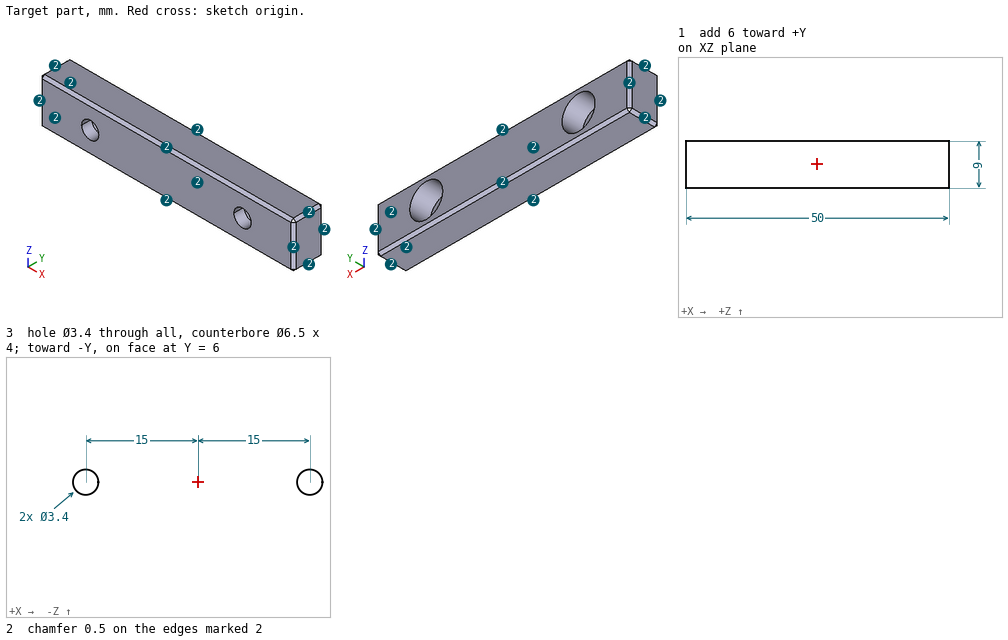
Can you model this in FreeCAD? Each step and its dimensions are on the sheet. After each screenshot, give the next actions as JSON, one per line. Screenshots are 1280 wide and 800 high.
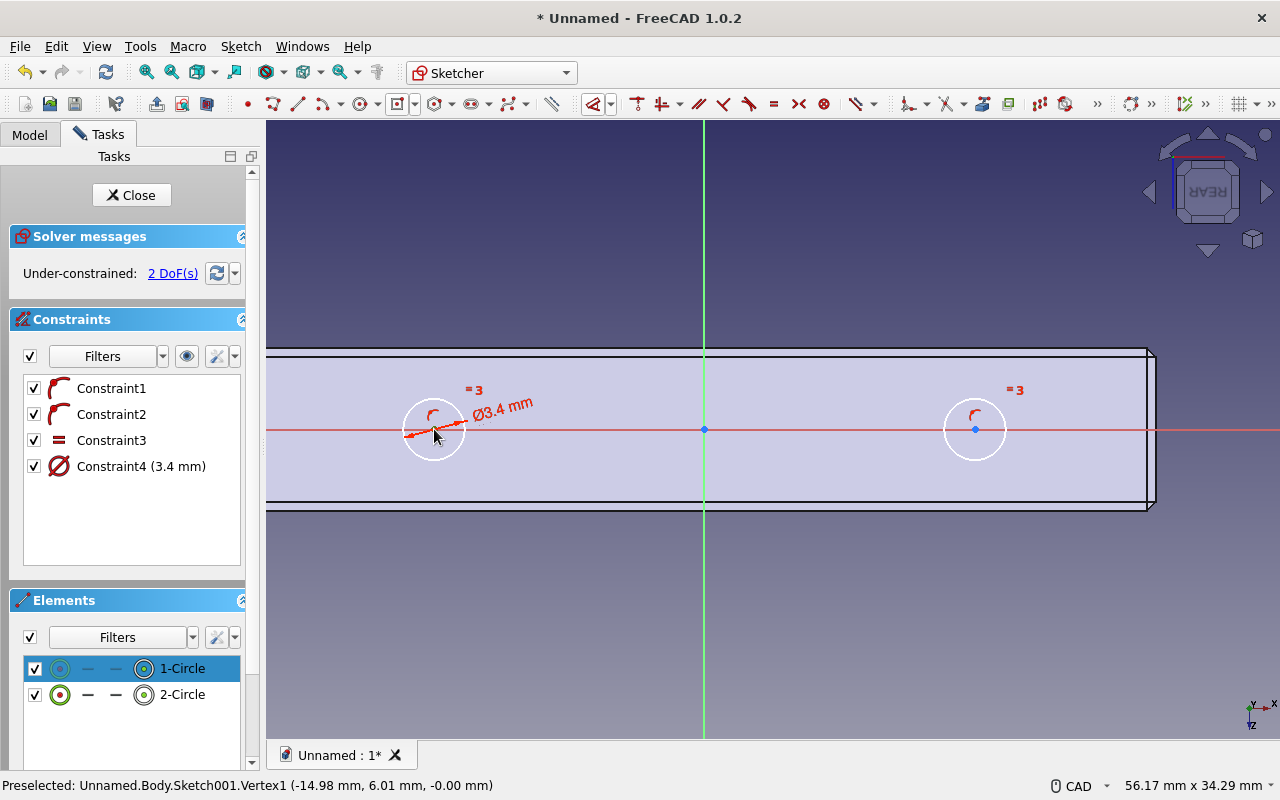
{"action": "left_click", "coordinate": [610, 104]}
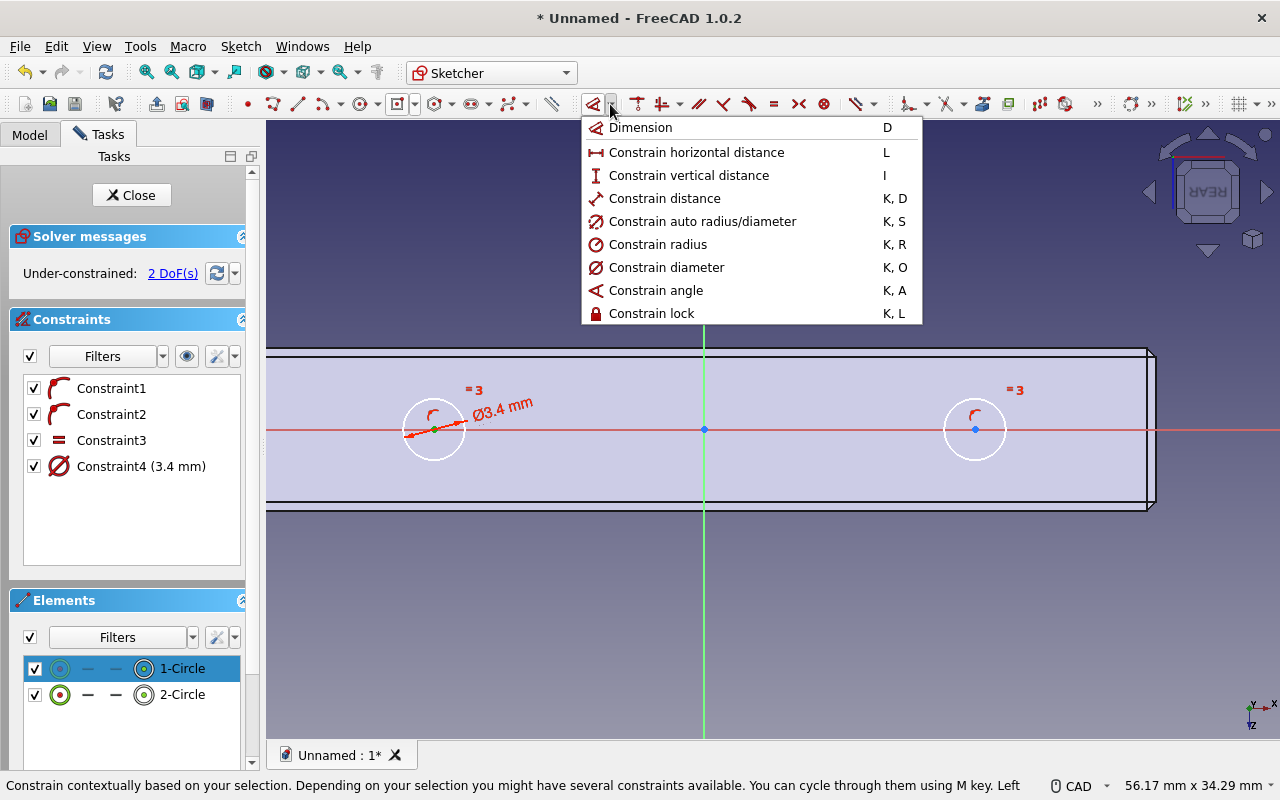
{"action": "left_click", "coordinate": [752, 152]}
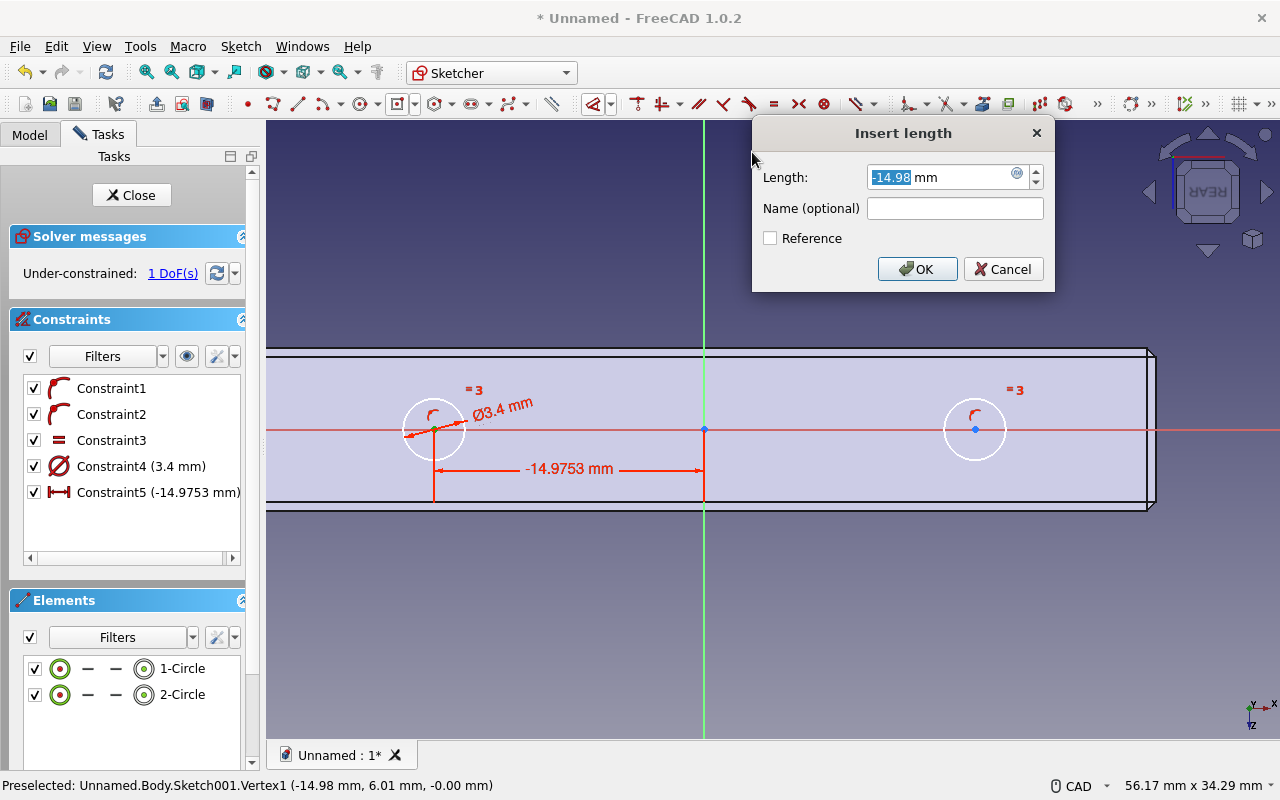
{"action": "type", "text": "-15"}
{"action": "key", "text": "Return"}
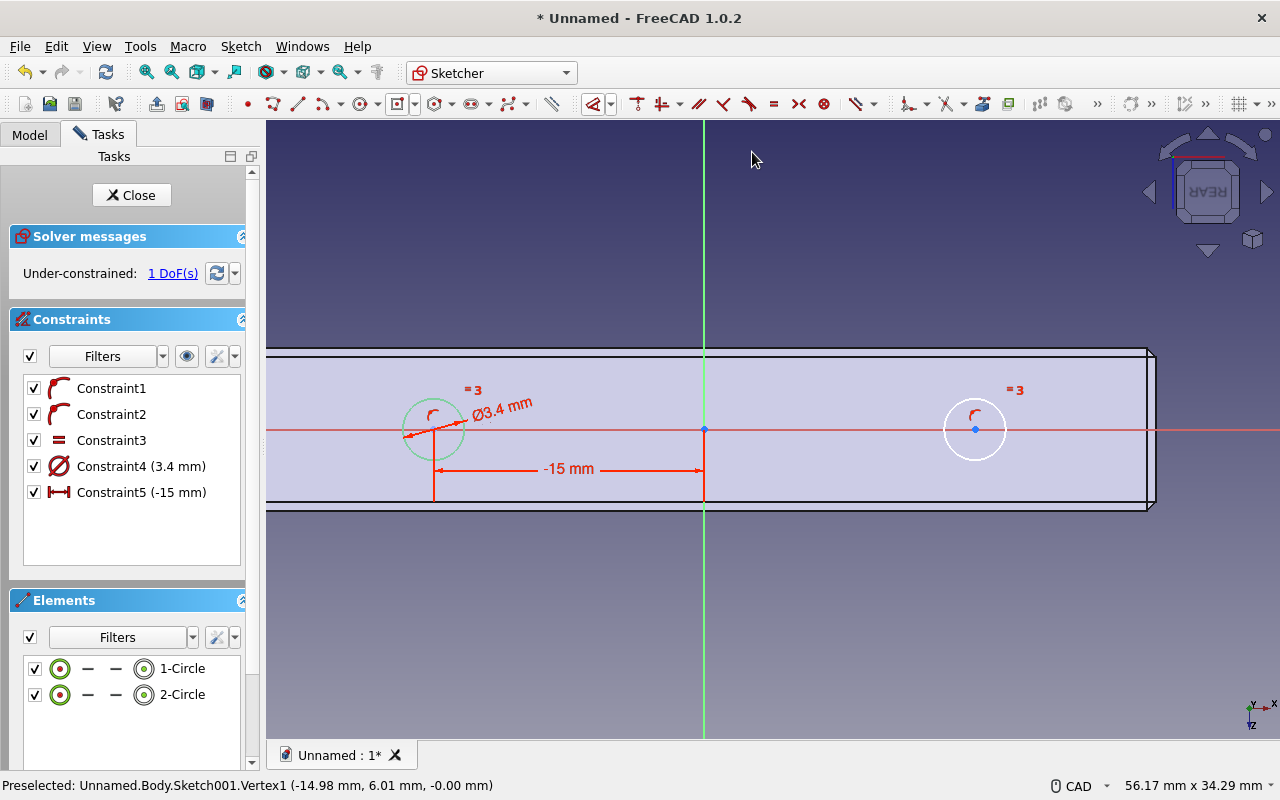
{"action": "left_click", "coordinate": [975, 429]}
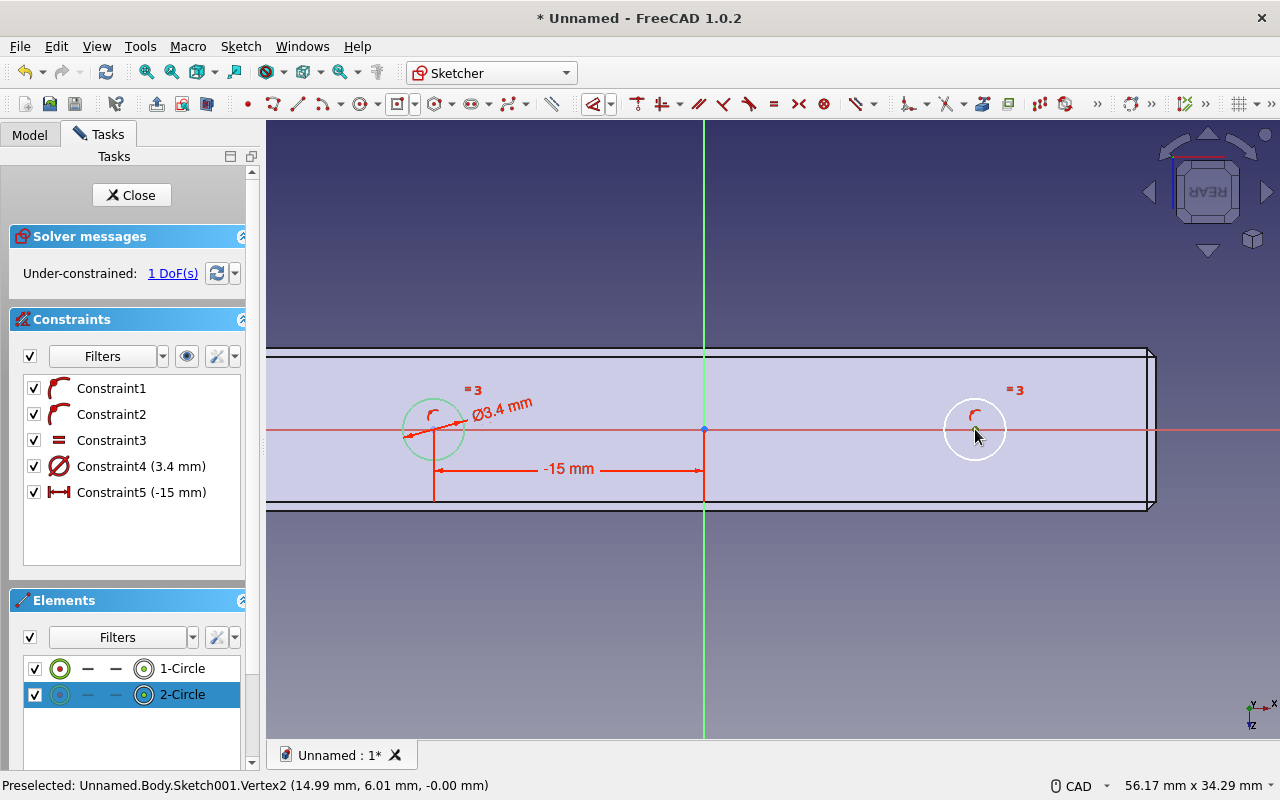
{"action": "key", "text": "l"}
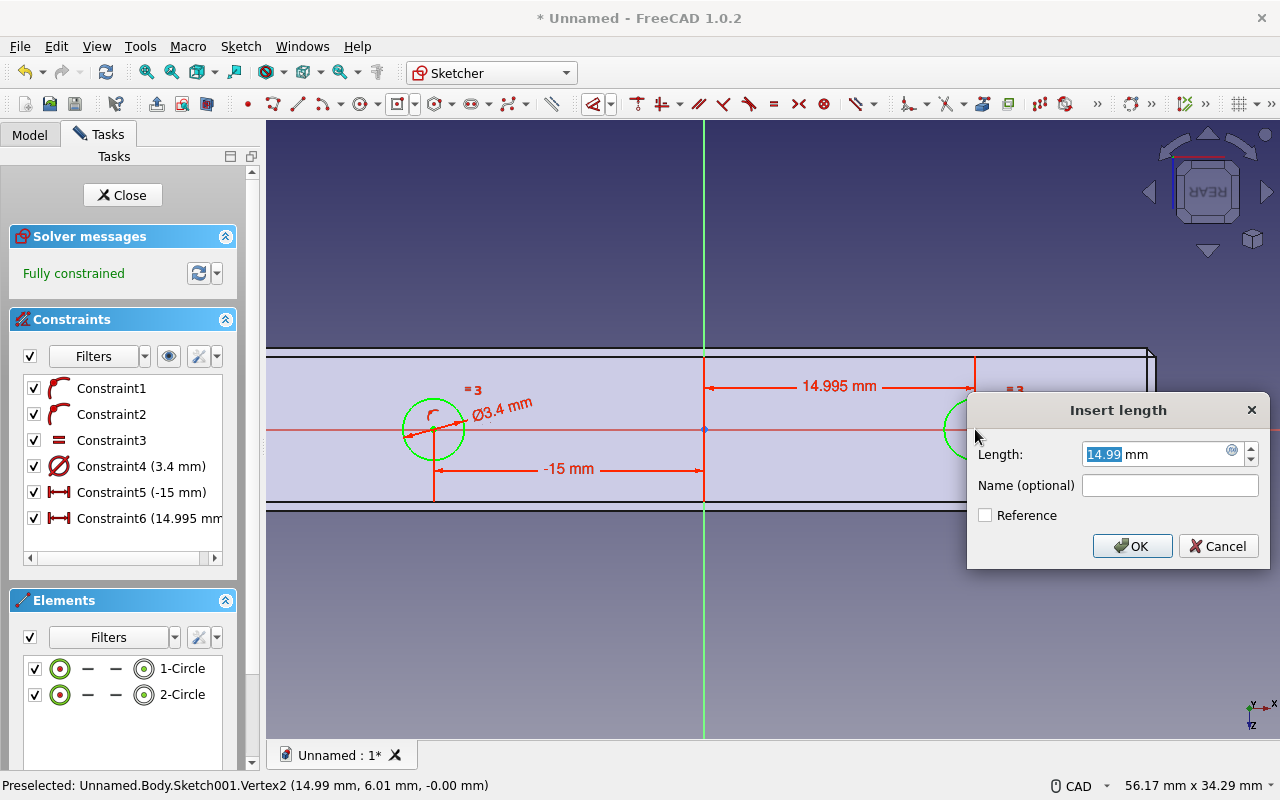
{"action": "type", "text": "15"}
{"action": "key", "text": "Return"}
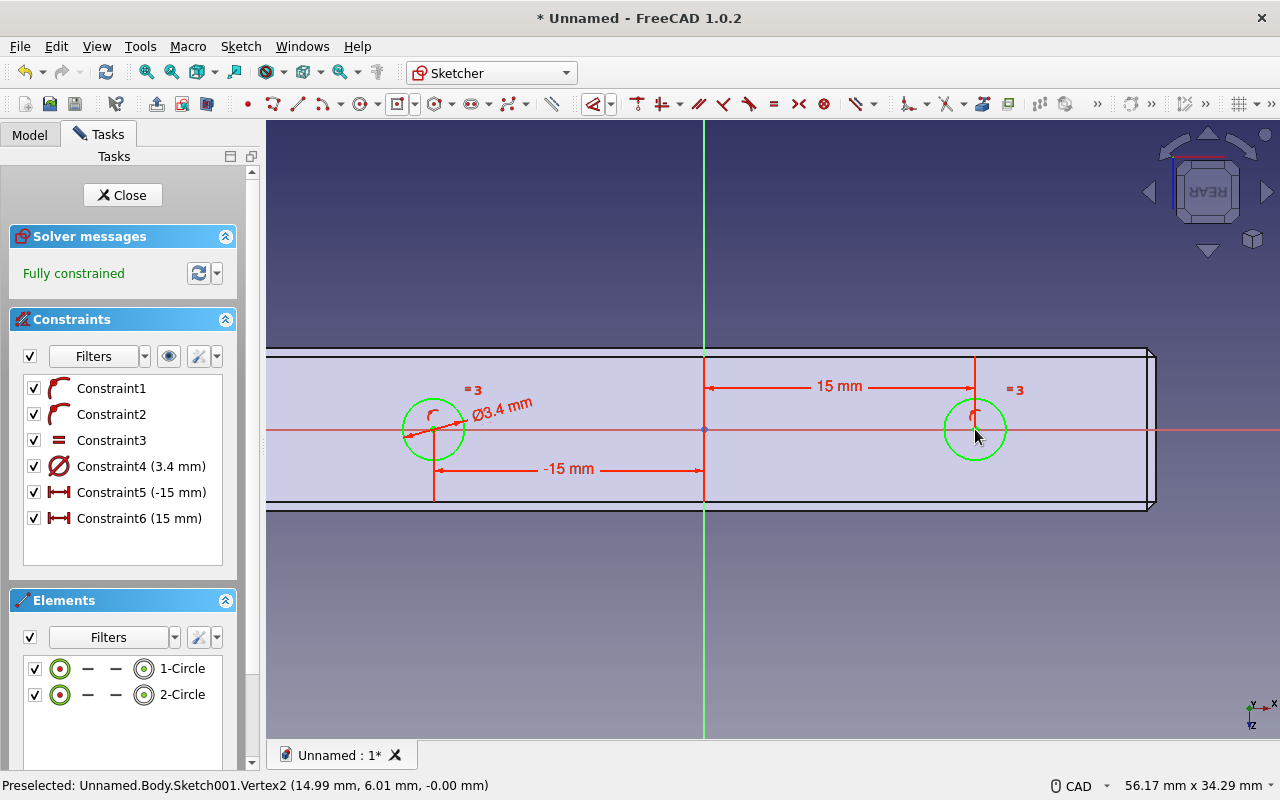
{"action": "left_click", "coordinate": [123, 195]}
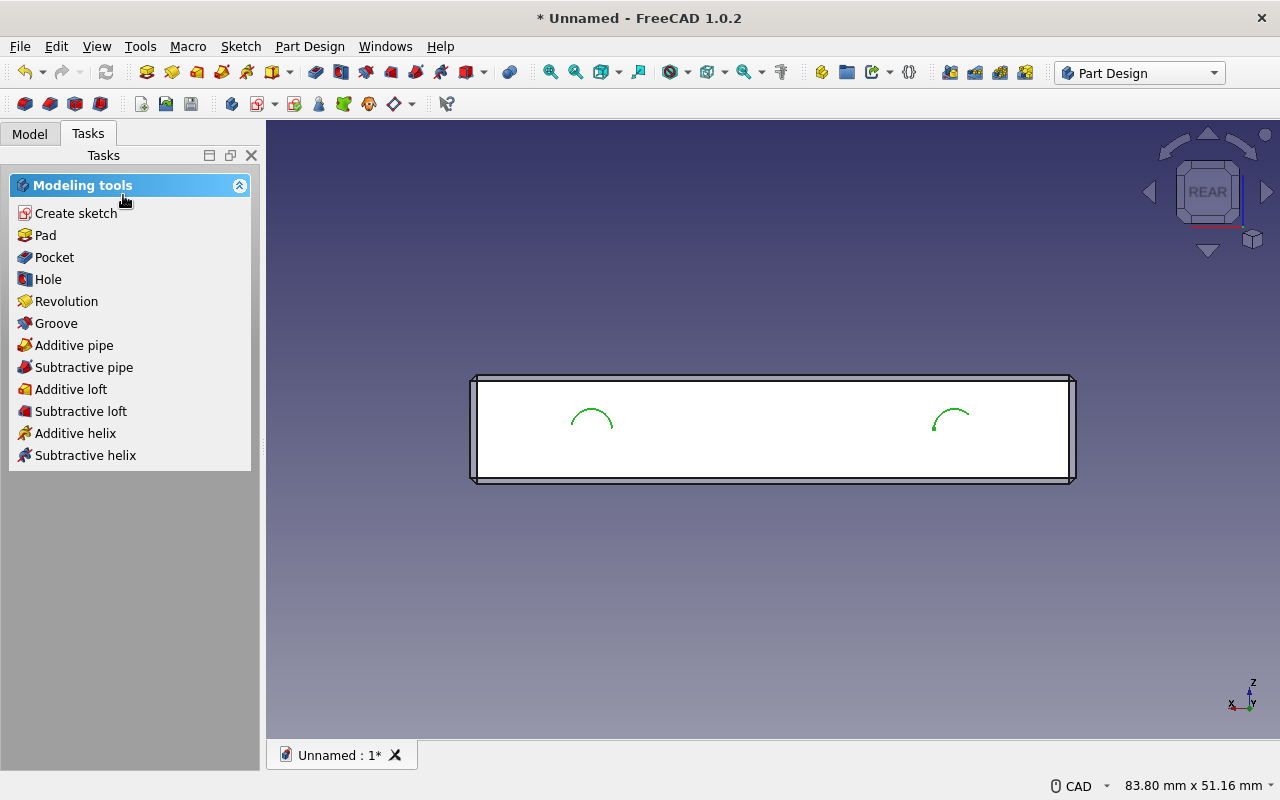
{"action": "left_click", "coordinate": [341, 72]}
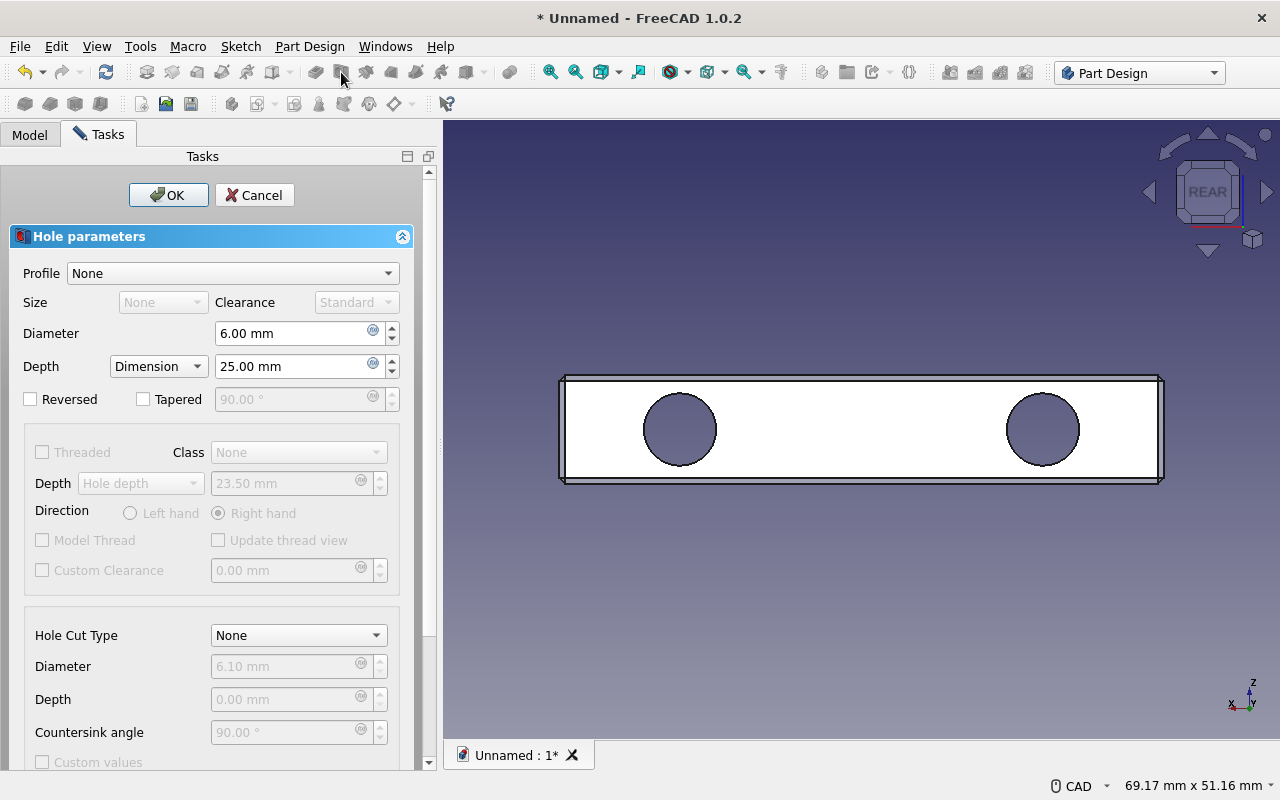
{"action": "triple_click", "coordinate": [300, 334]}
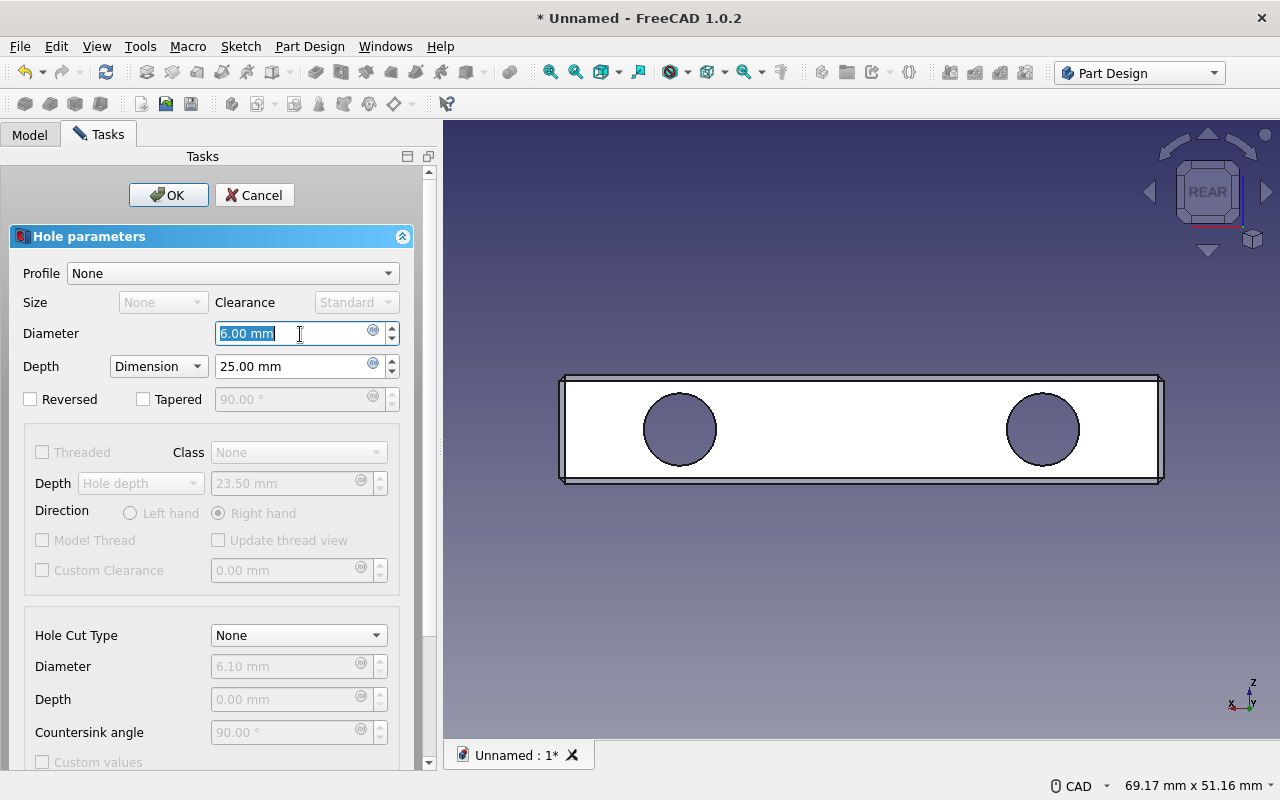
{"action": "type", "text": "3.4"}
{"action": "key", "text": "Tab"}